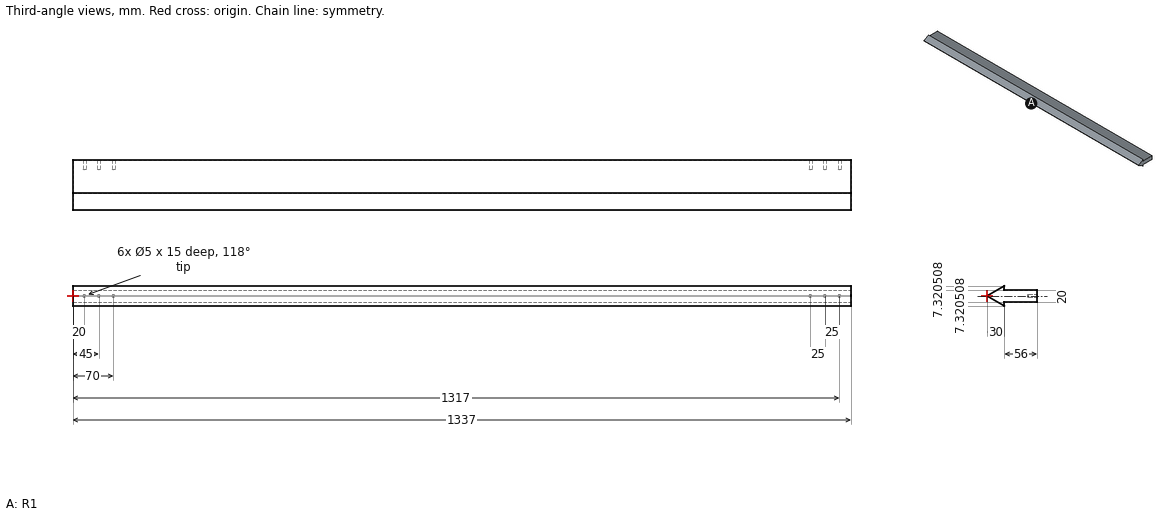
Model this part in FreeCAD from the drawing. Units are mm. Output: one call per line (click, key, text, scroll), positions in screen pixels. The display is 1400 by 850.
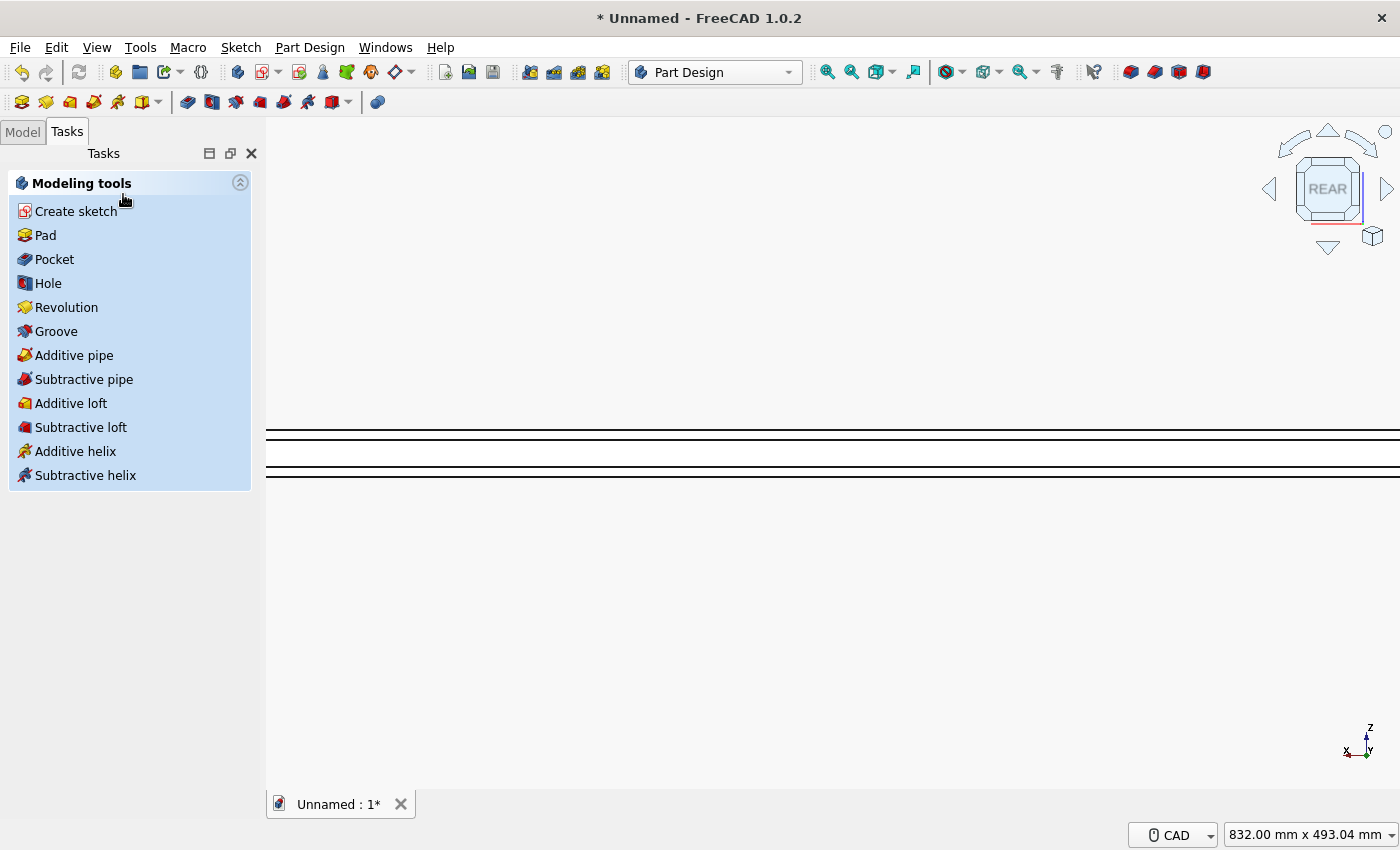
click(212, 102)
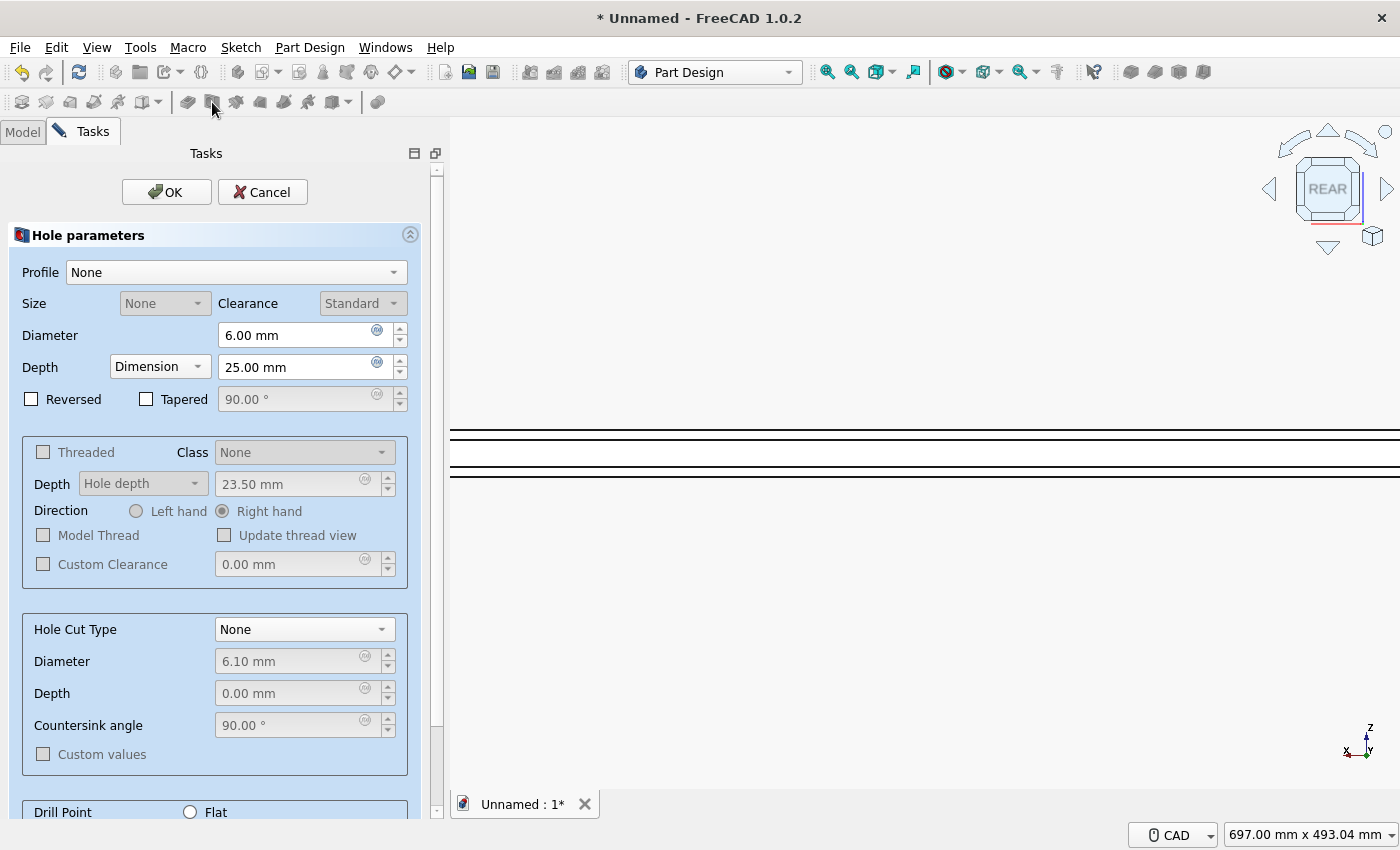
triple_click(305, 335)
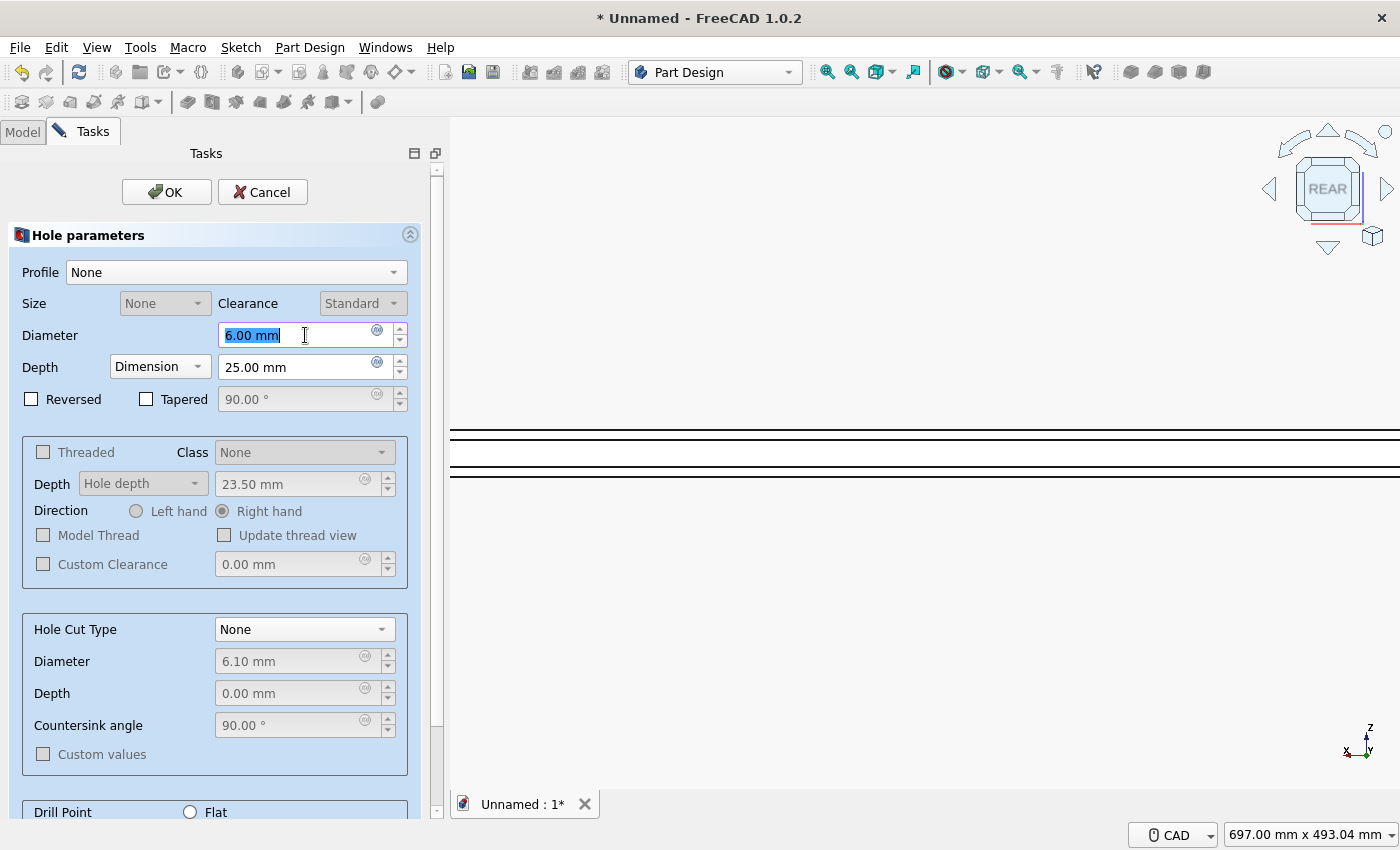
text(5)
key(Tab)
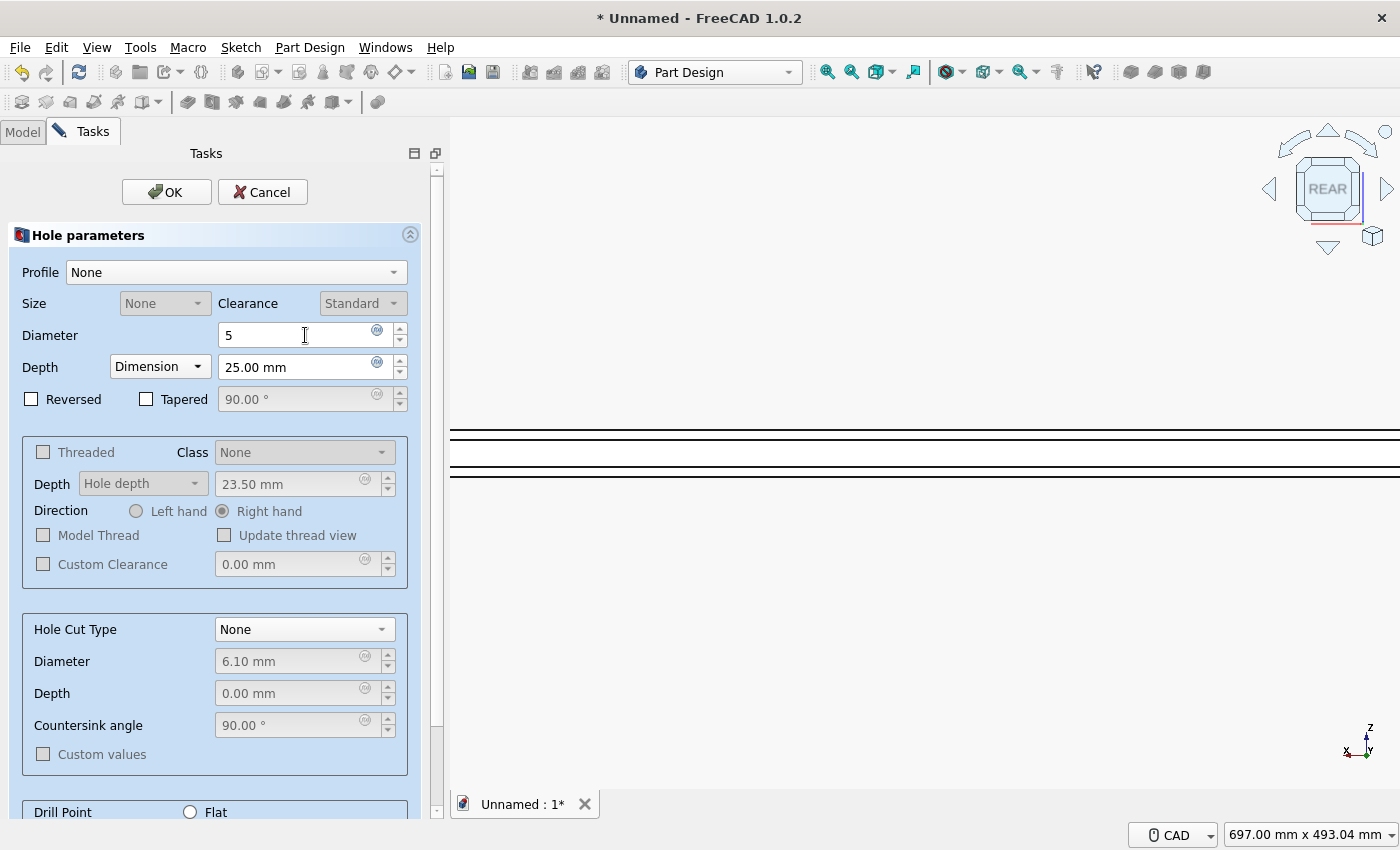
triple_click(305, 367)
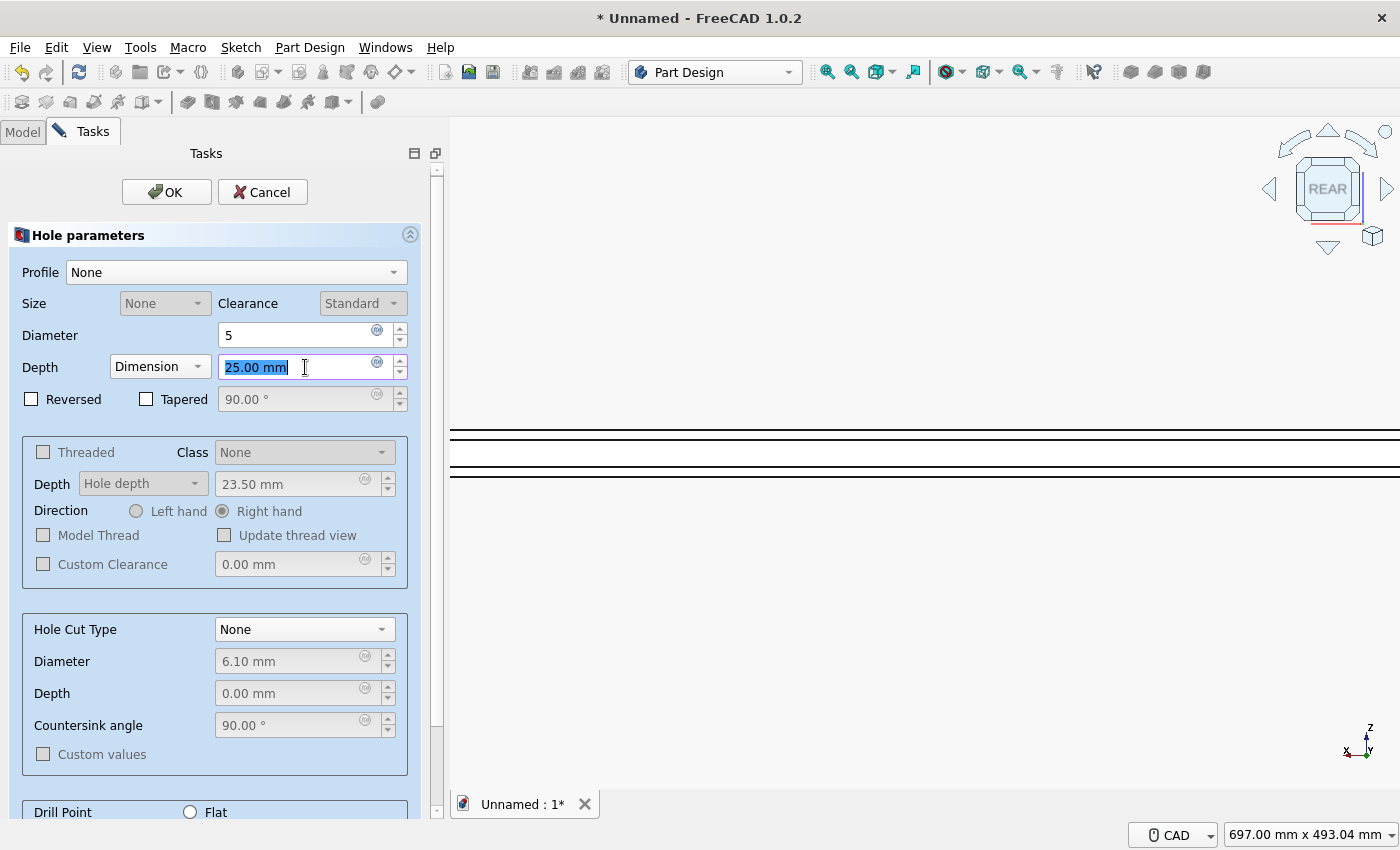
text(15)
key(Tab)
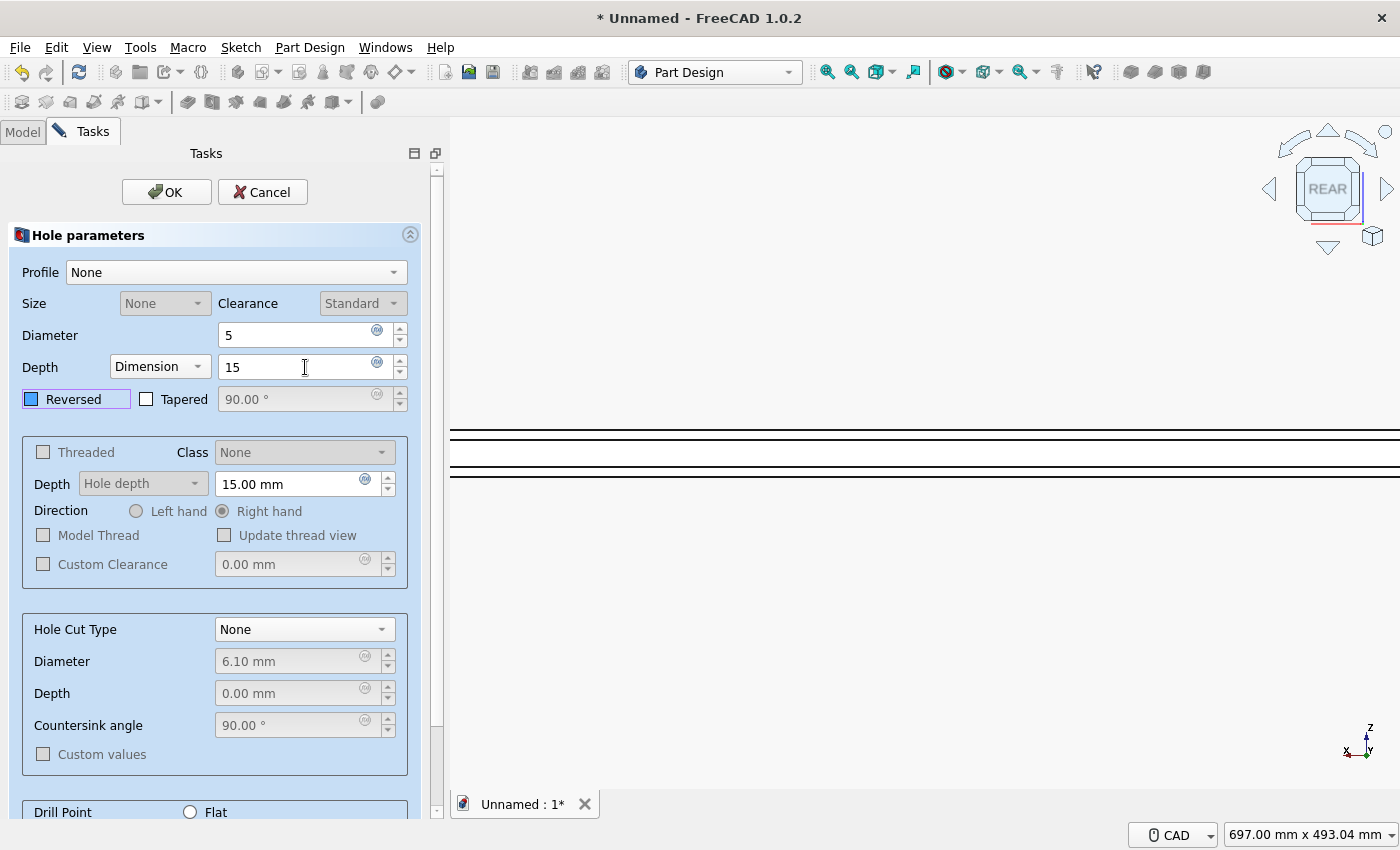
click(167, 192)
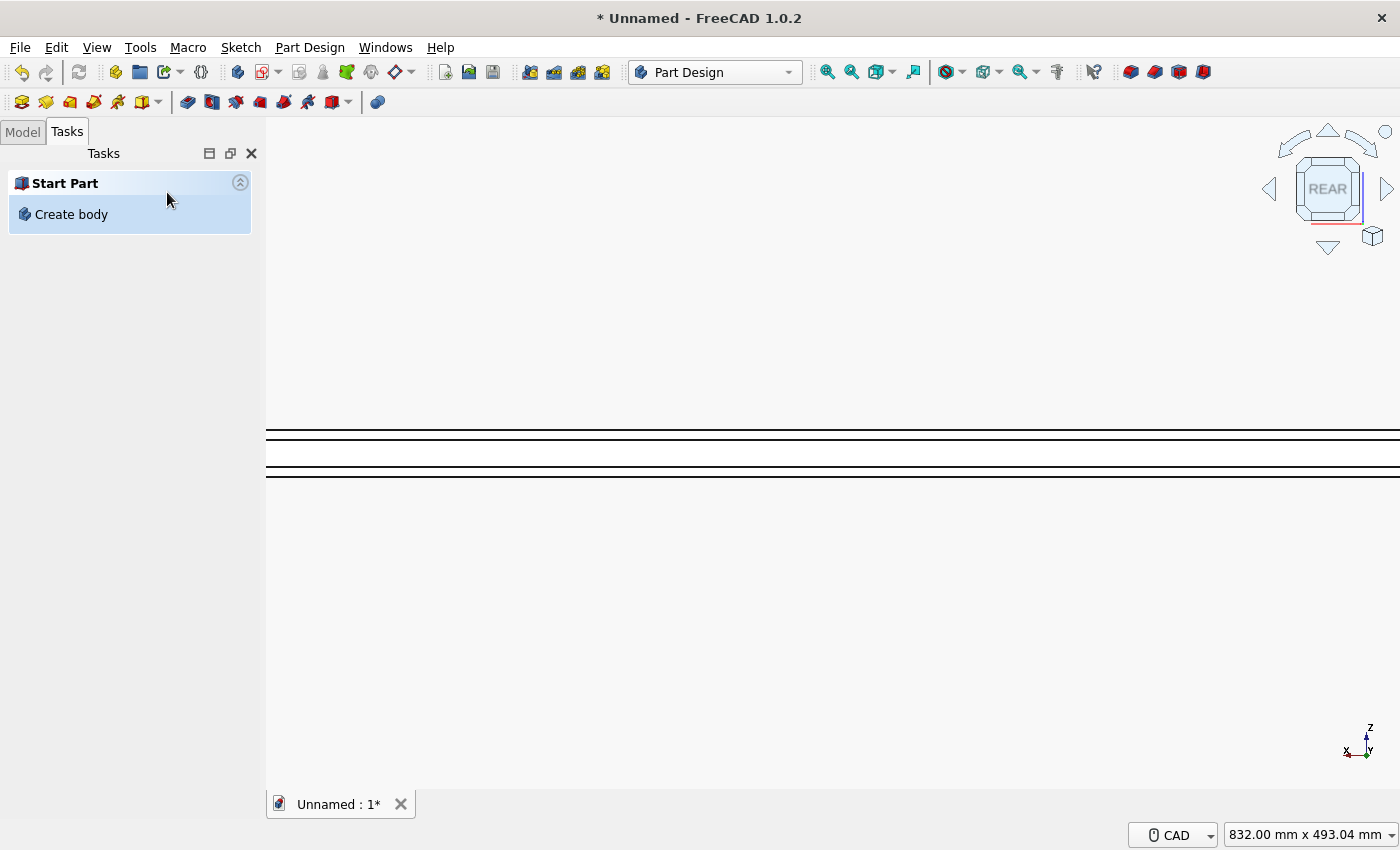
key(0)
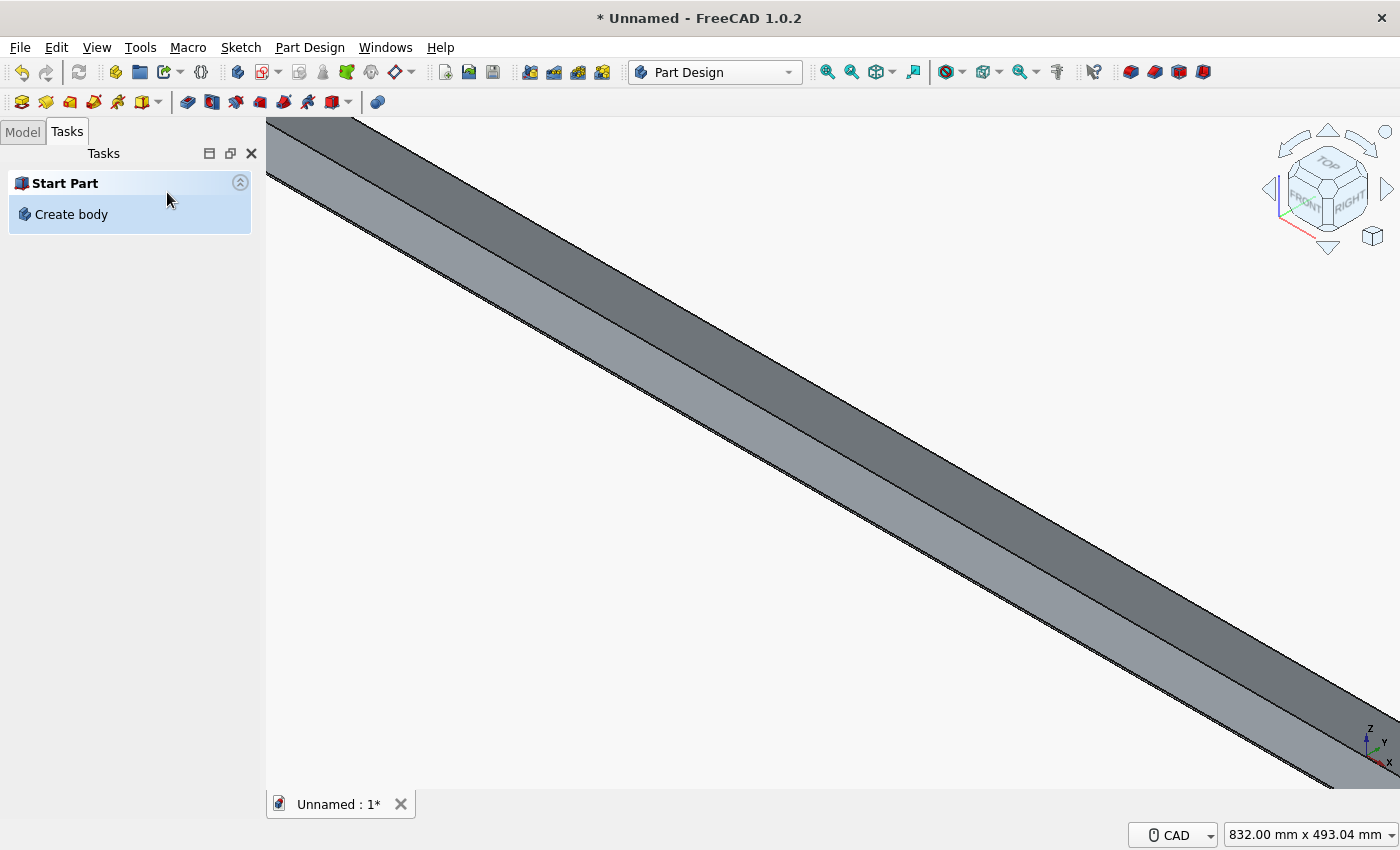
click(828, 72)